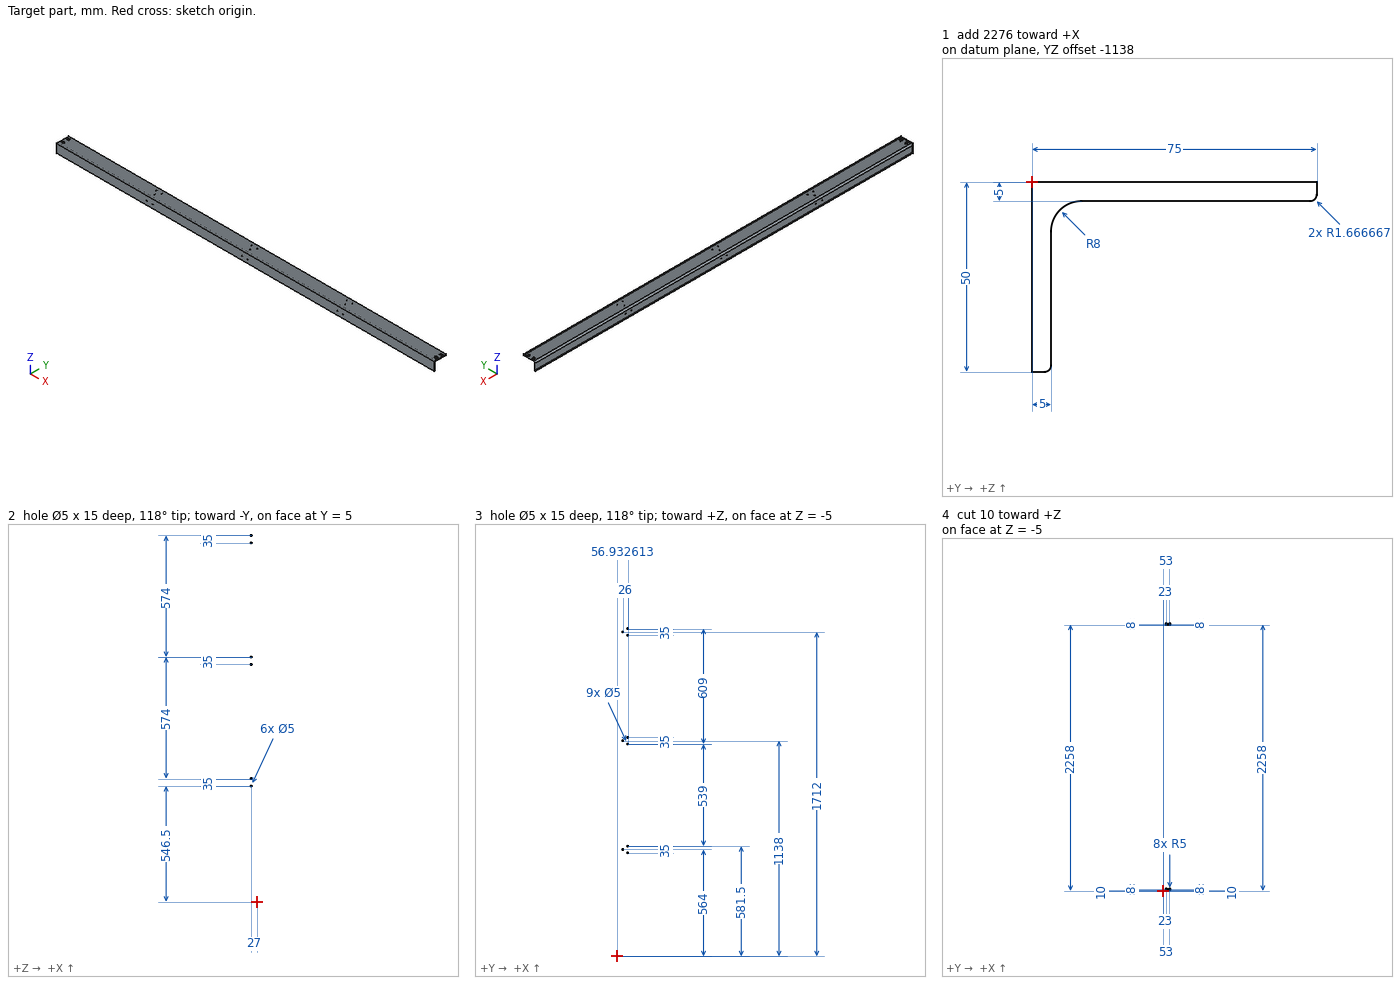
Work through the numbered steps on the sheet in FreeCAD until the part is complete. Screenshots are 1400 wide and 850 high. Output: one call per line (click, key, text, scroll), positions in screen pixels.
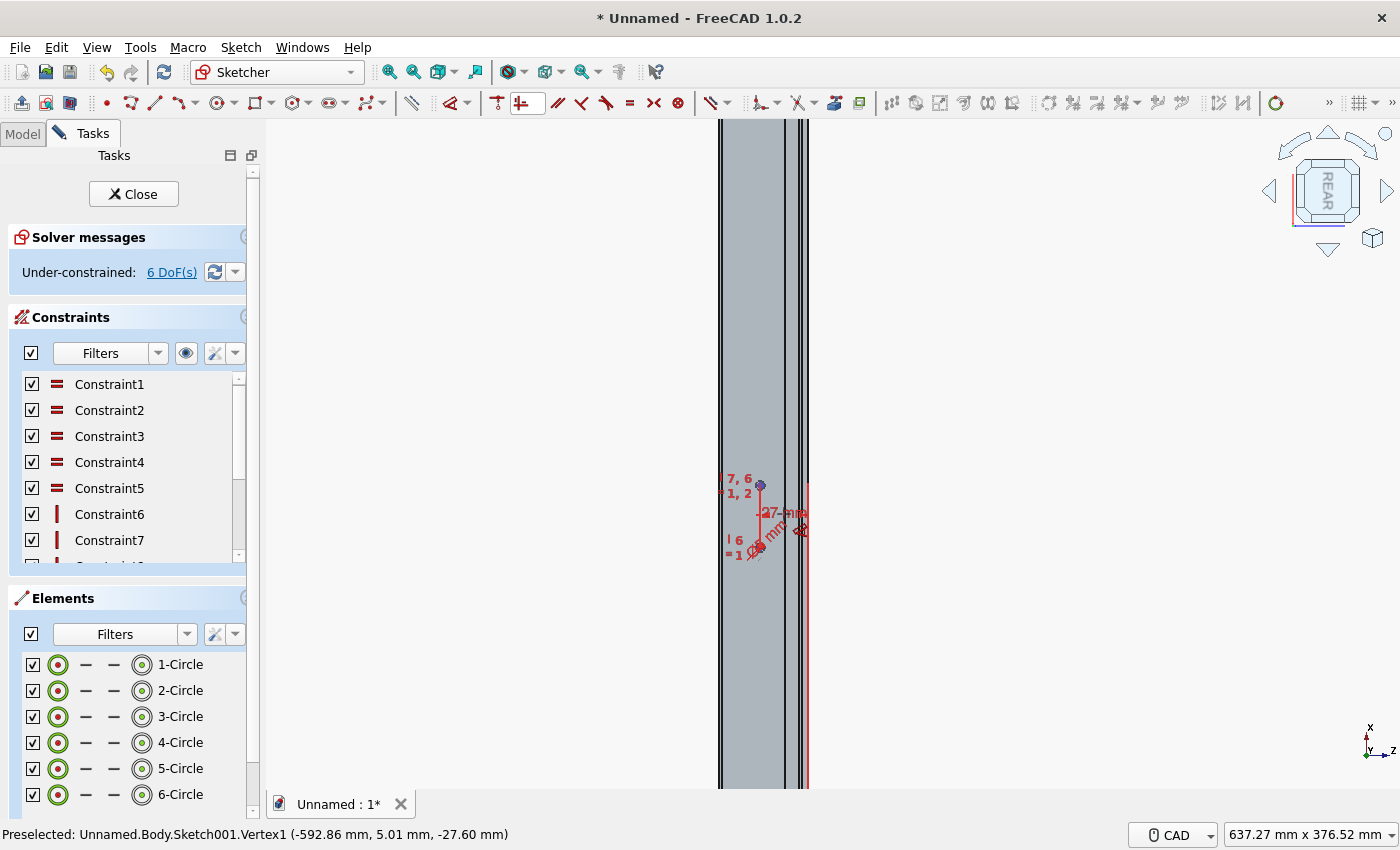
click(760, 548)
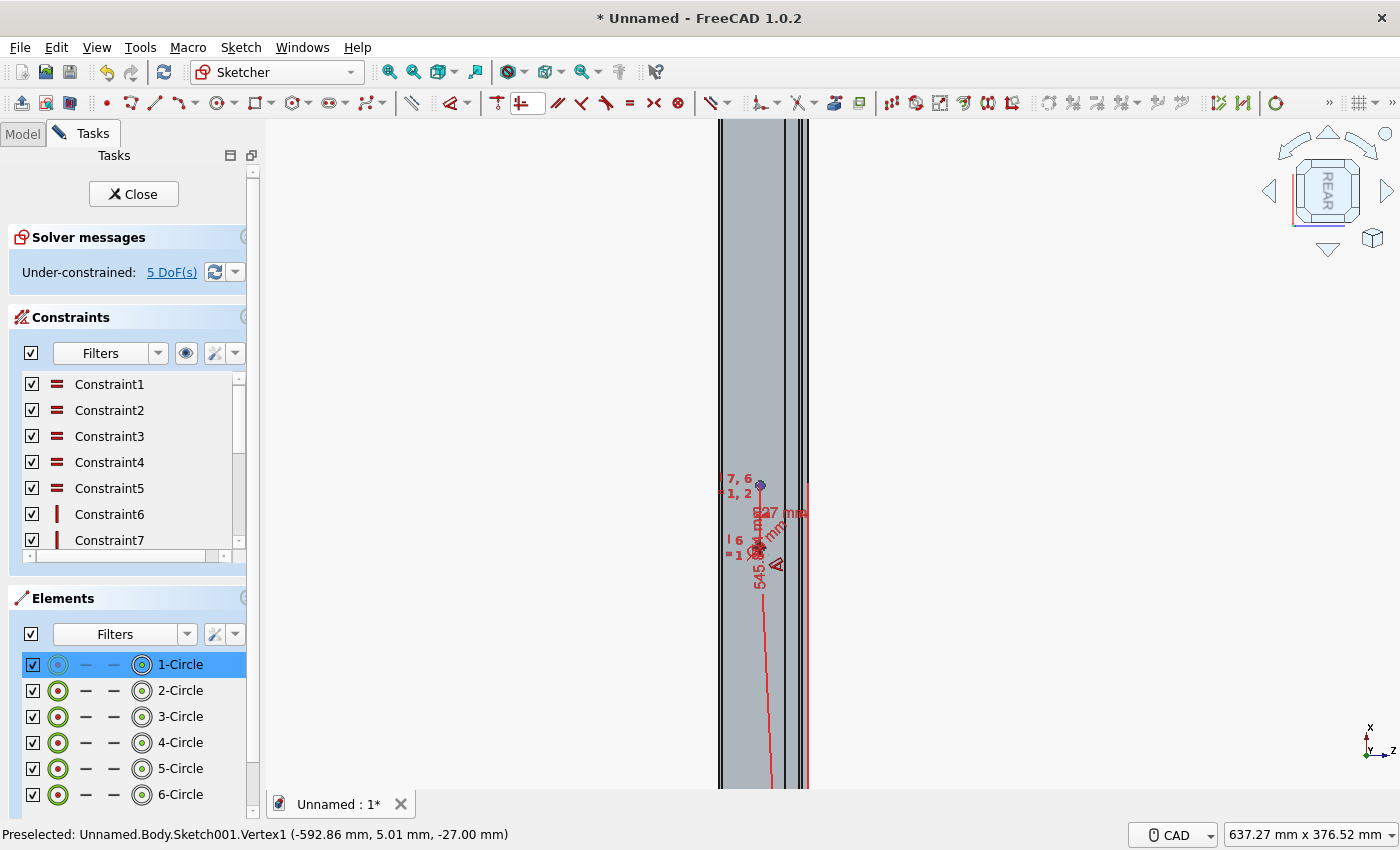
click(760, 485)
click(702, 517)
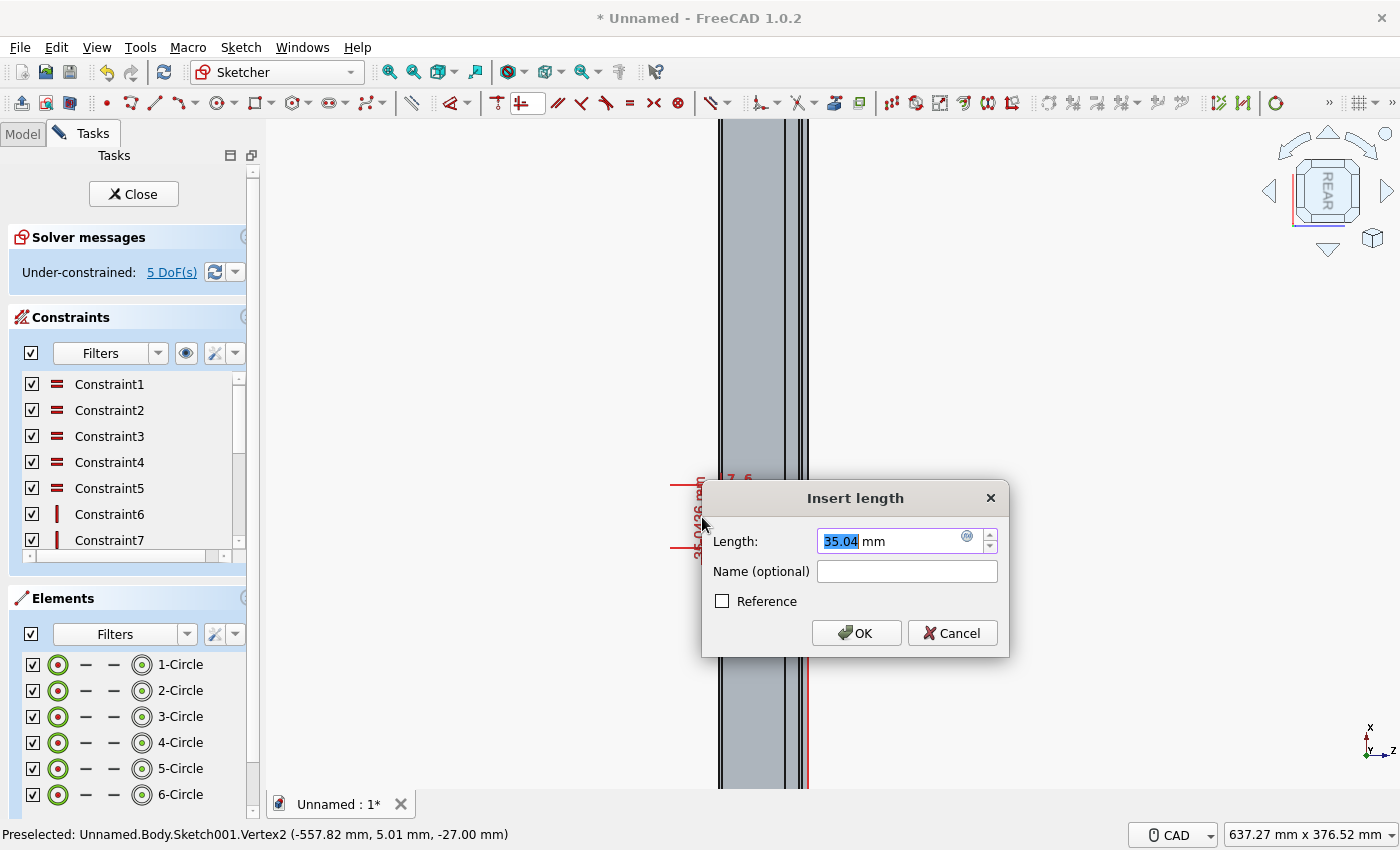
text(35)
key(Return)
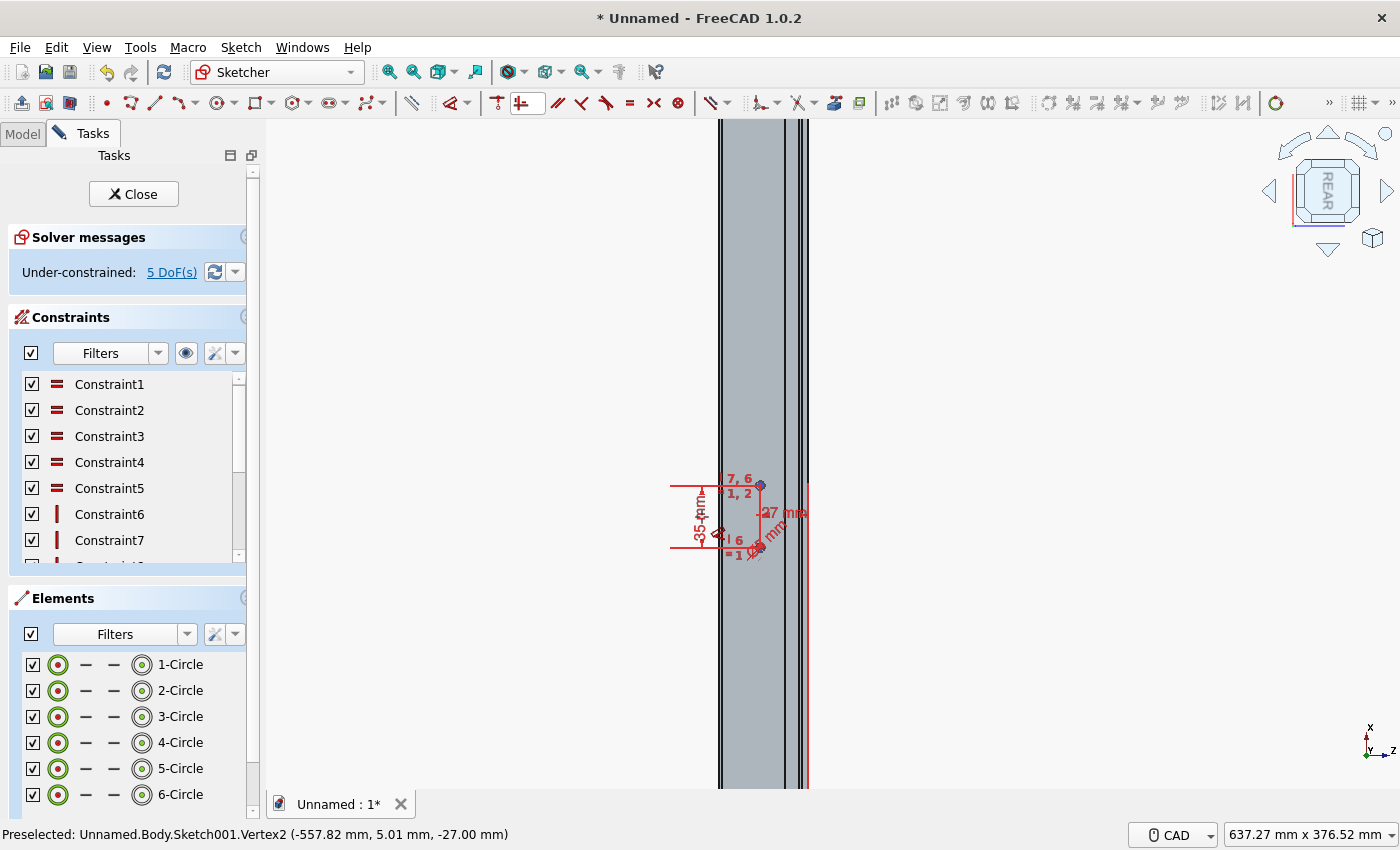
scroll(762, 529, down, 10)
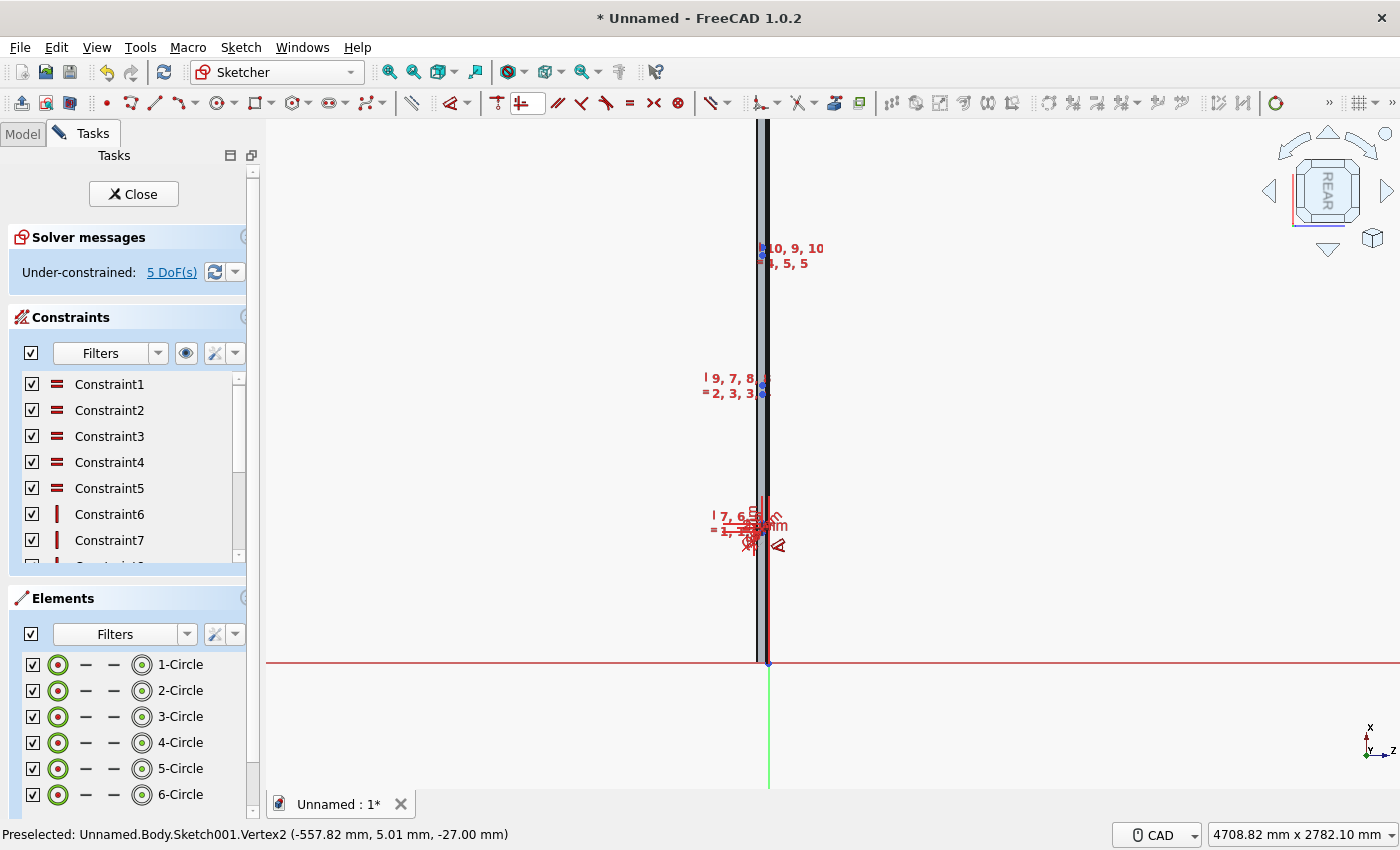
scroll(762, 385, up, 8)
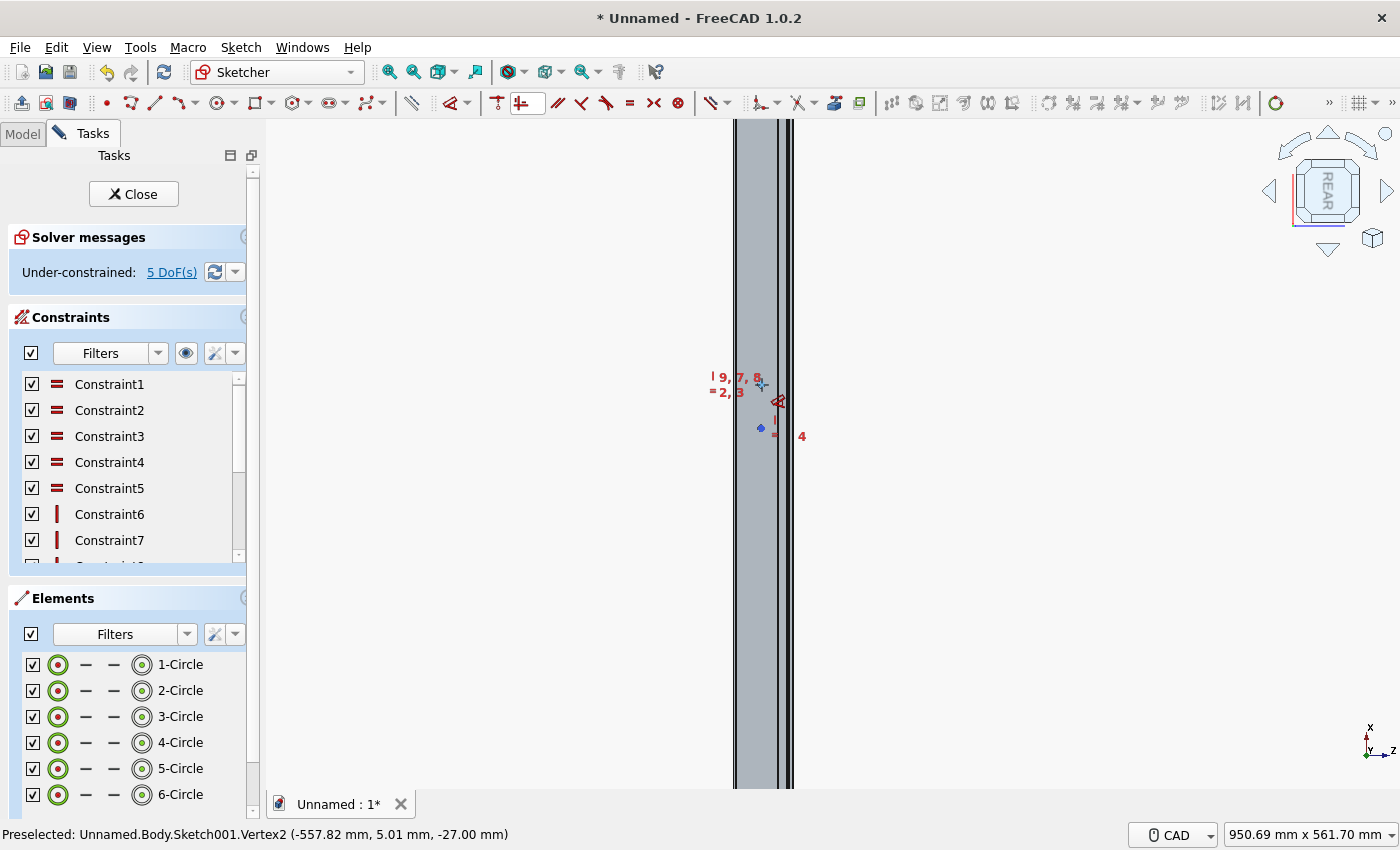
click(761, 385)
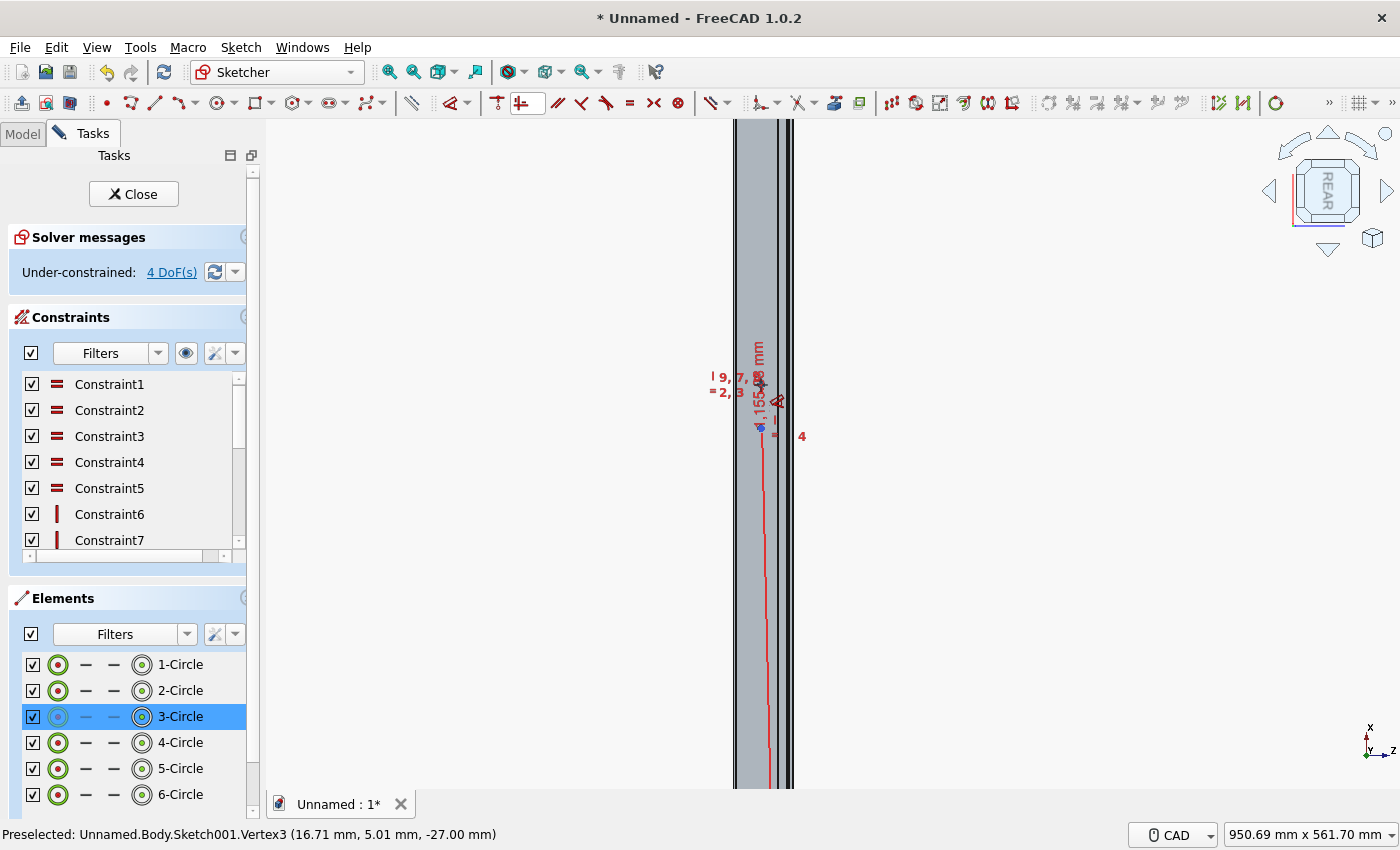
click(761, 428)
click(727, 407)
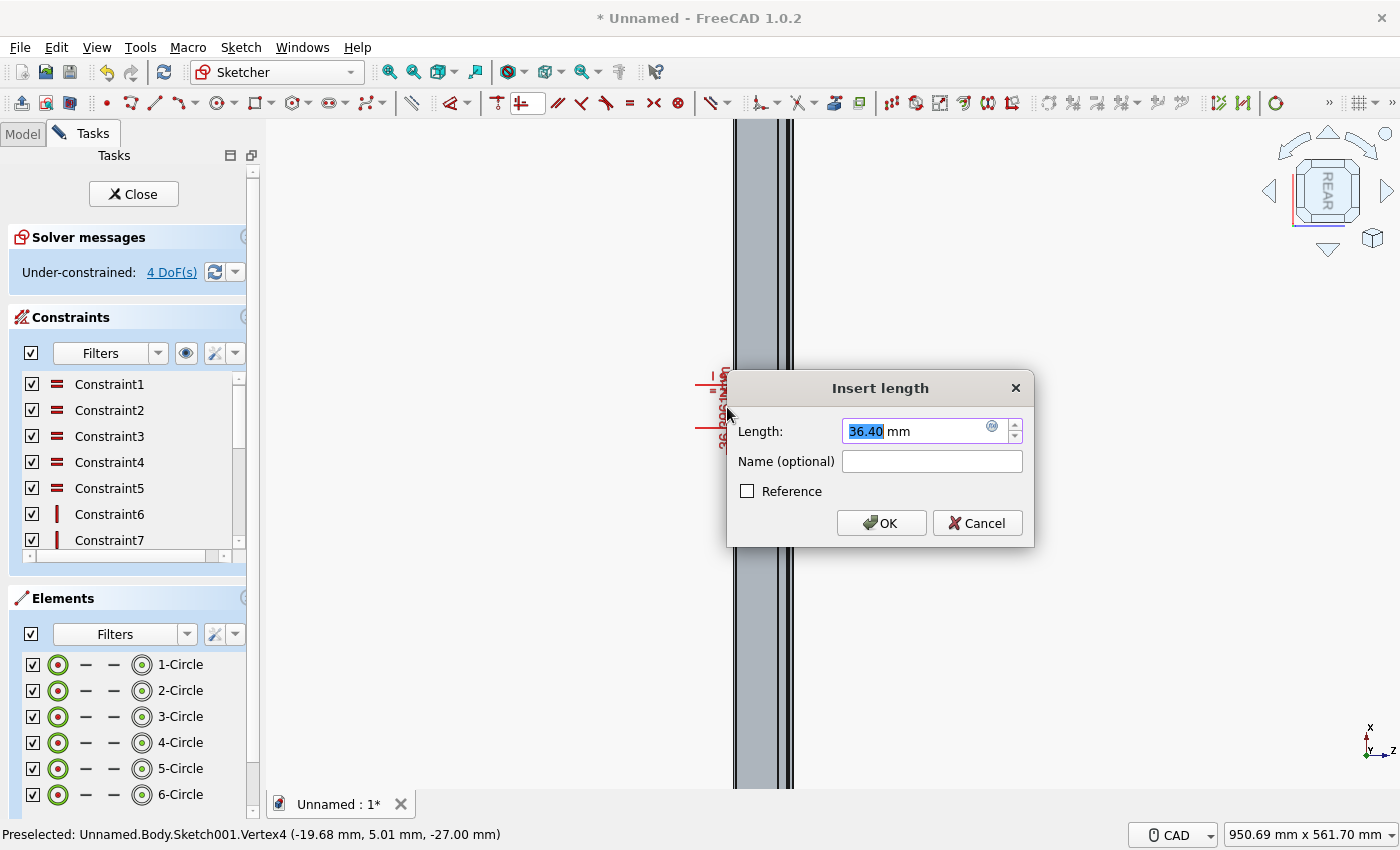
text(35)
key(Return)